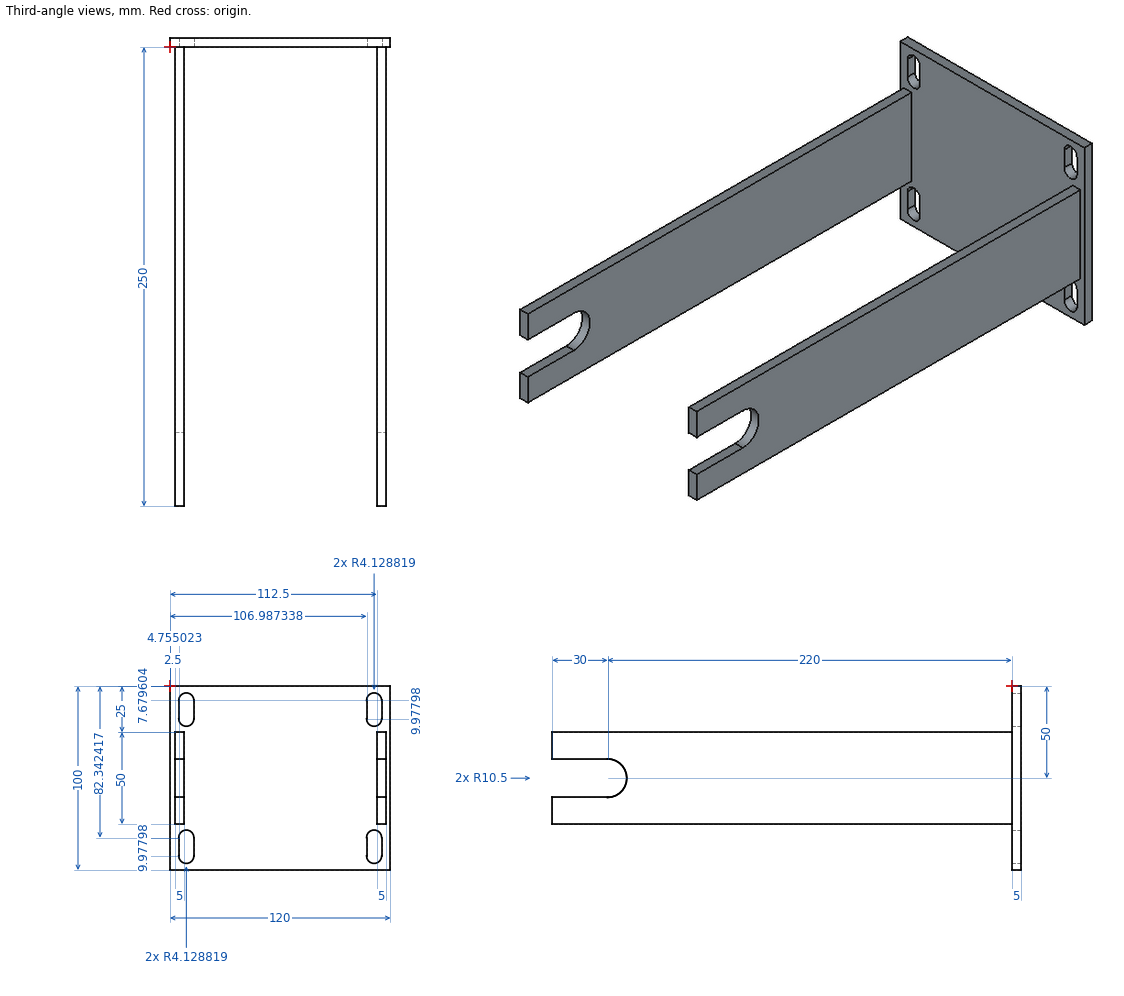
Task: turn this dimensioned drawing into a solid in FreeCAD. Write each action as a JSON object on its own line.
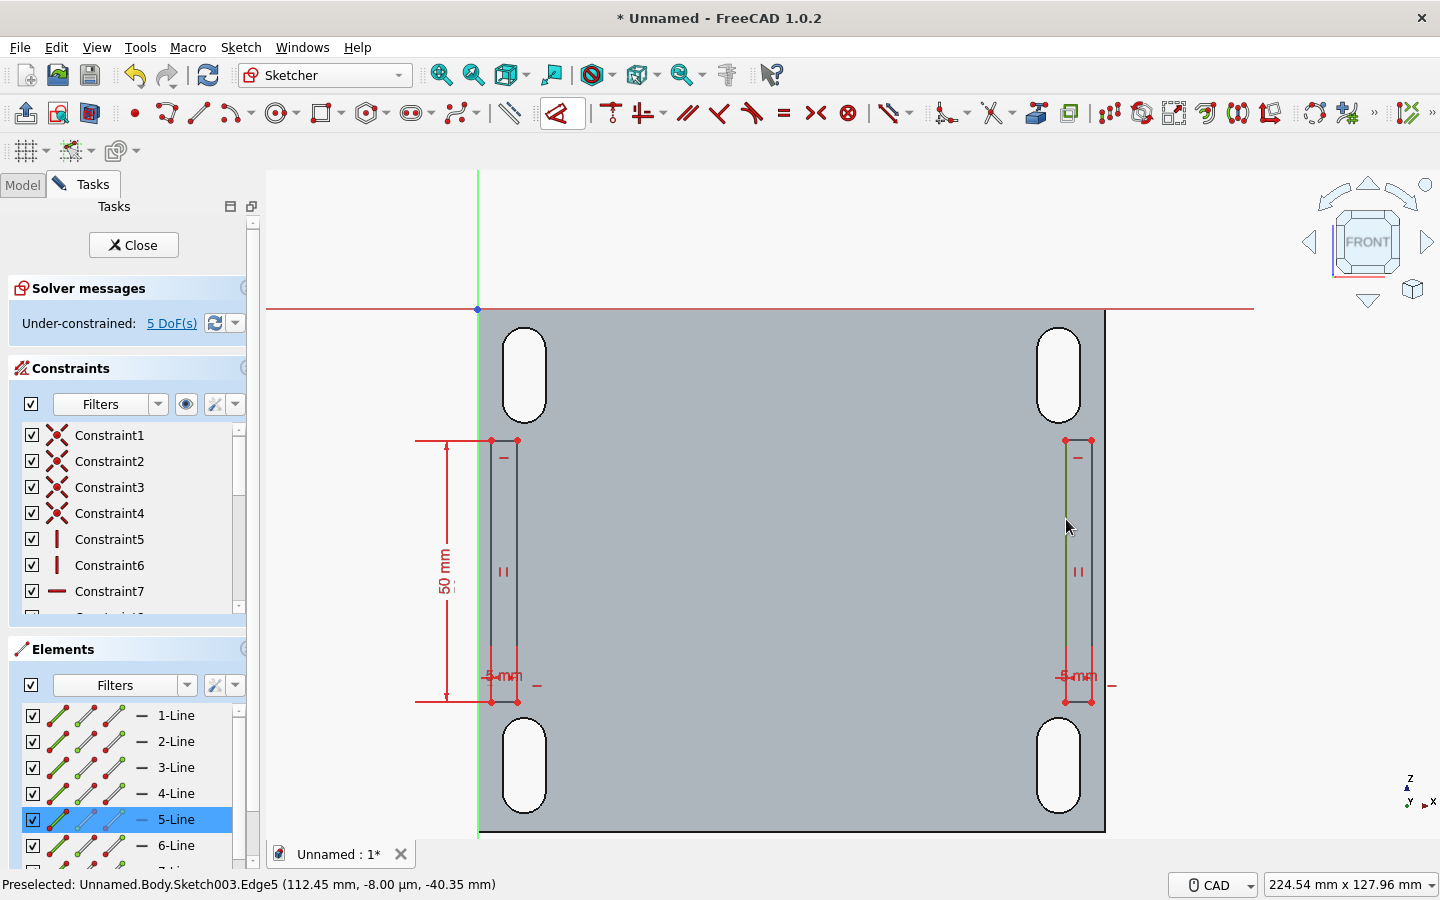
{"action": "key", "text": "i"}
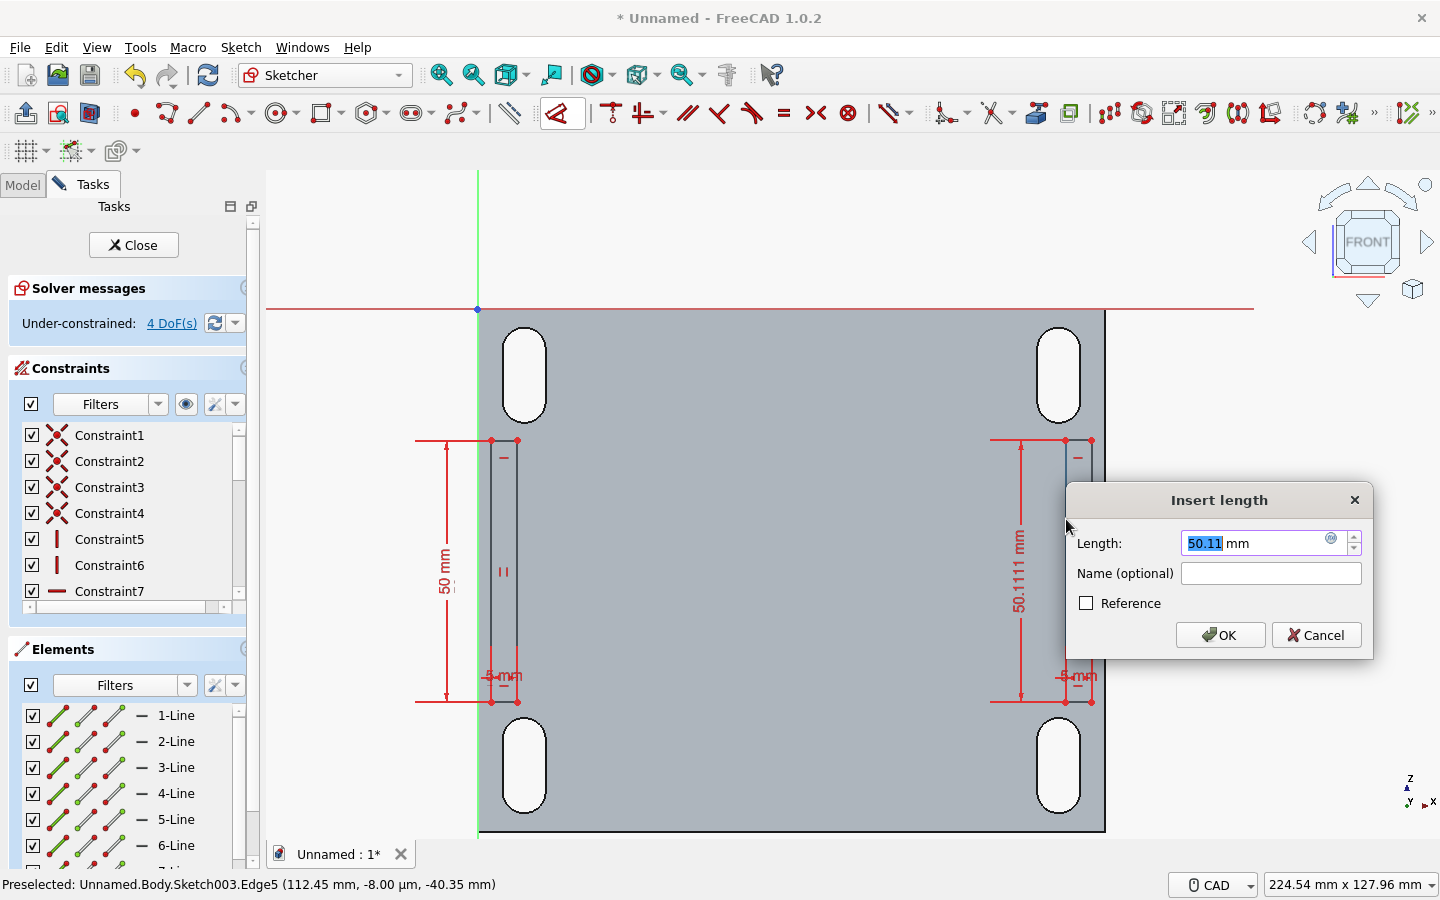
{"action": "type", "text": "50"}
{"action": "key", "text": "Return"}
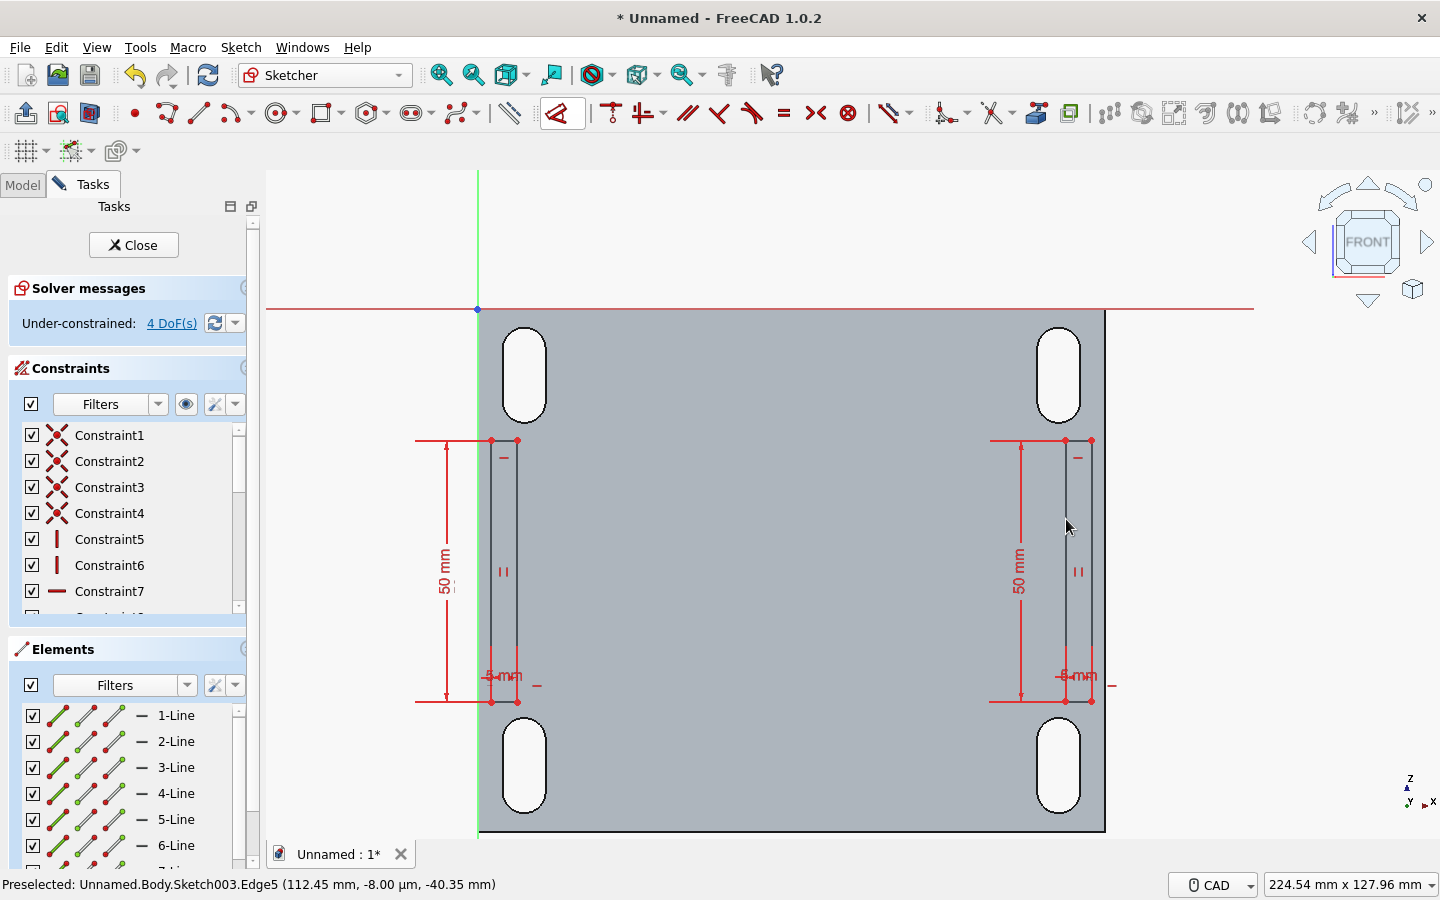
{"action": "left_click", "coordinate": [491, 441]}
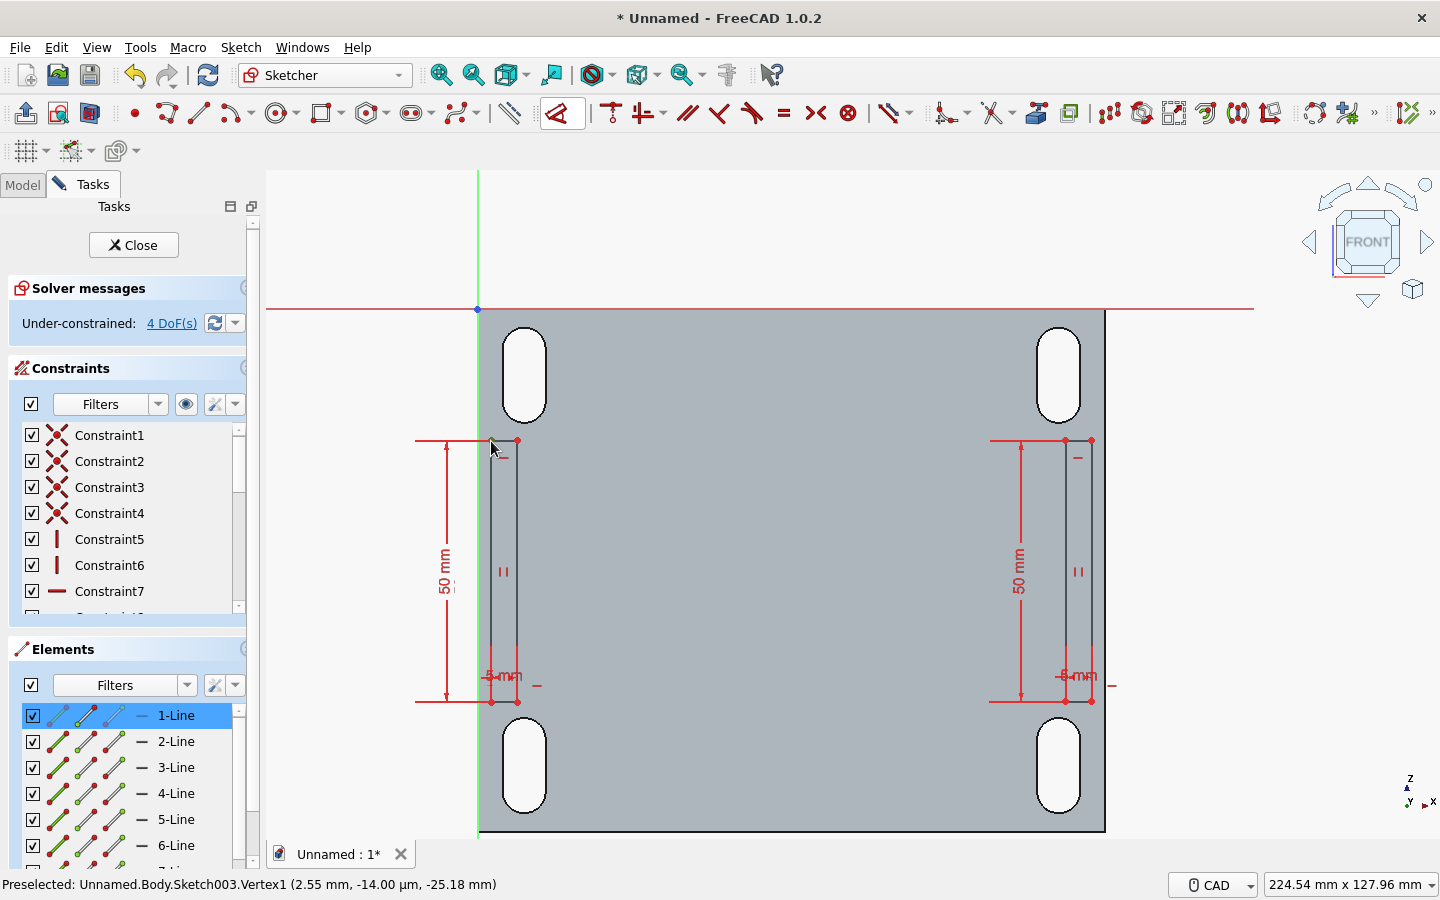
{"action": "key", "text": "i"}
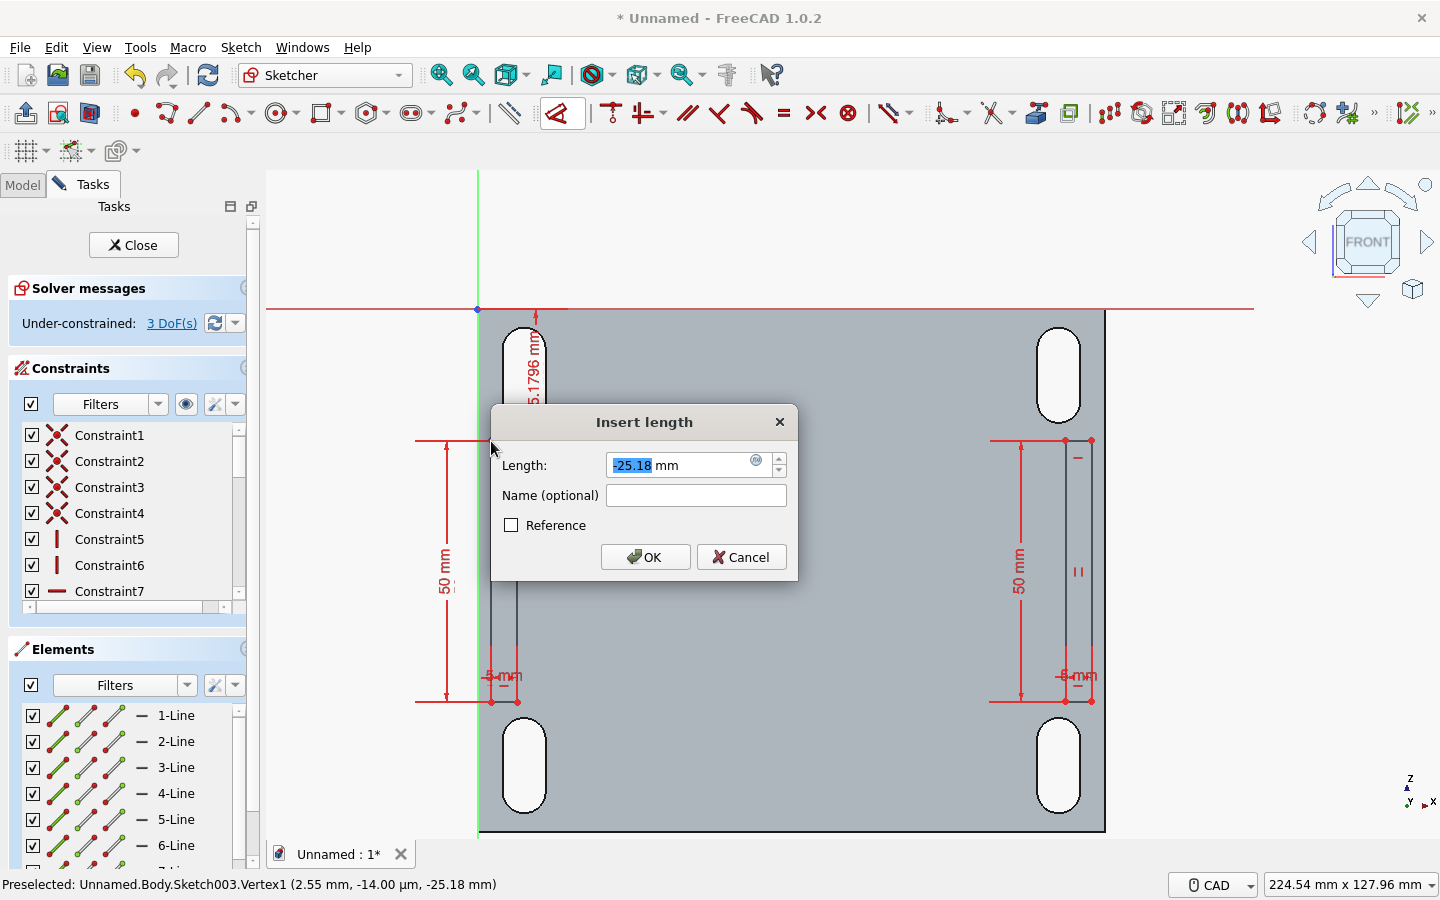
{"action": "type", "text": "-25"}
{"action": "key", "text": "Return"}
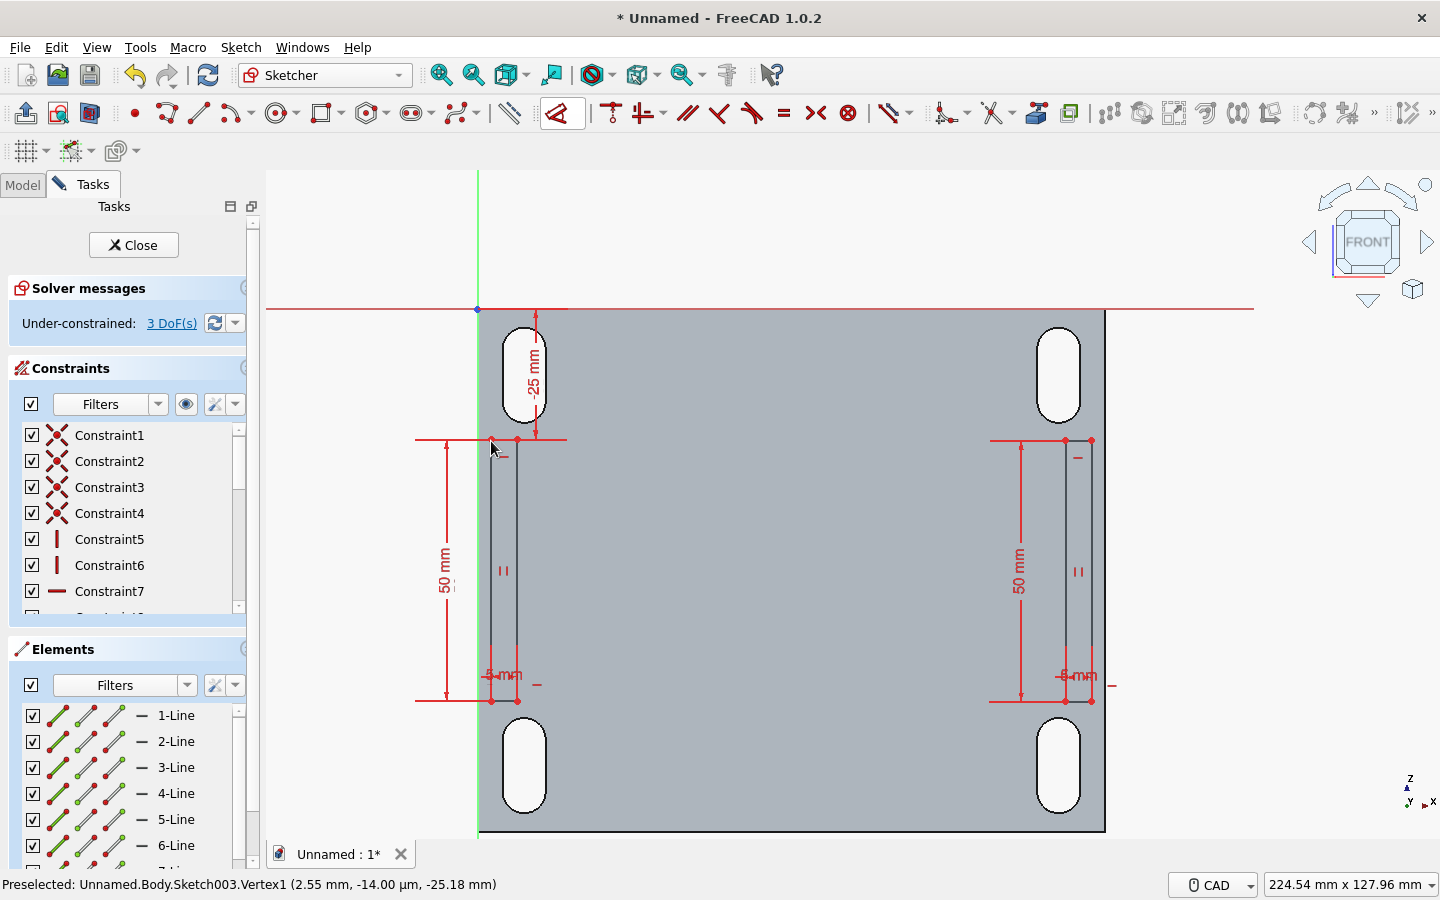
{"action": "left_click", "coordinate": [1066, 441]}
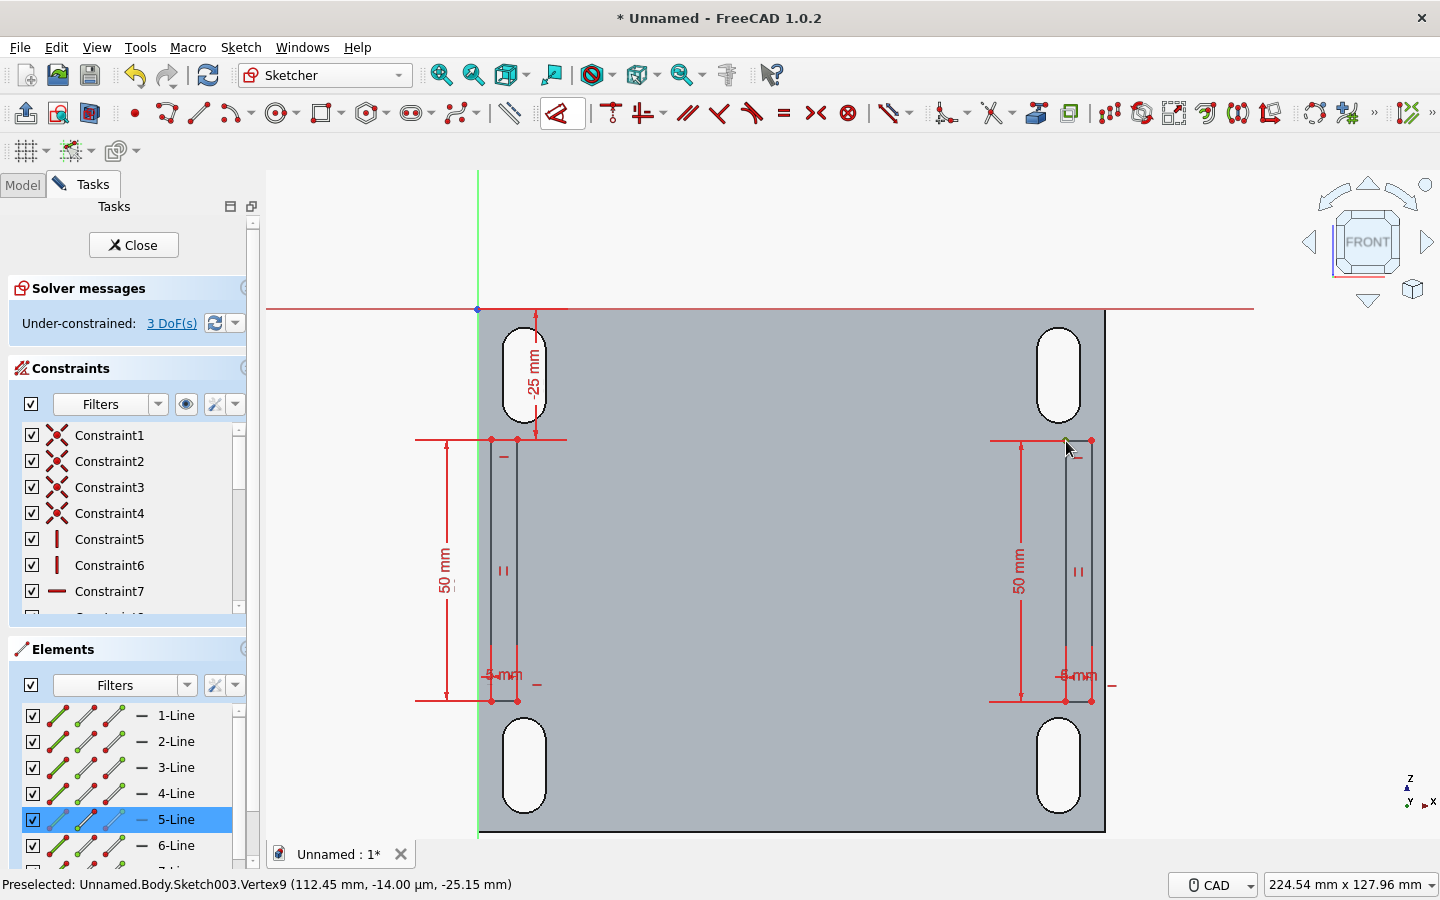
{"action": "left_click", "coordinate": [580, 114]}